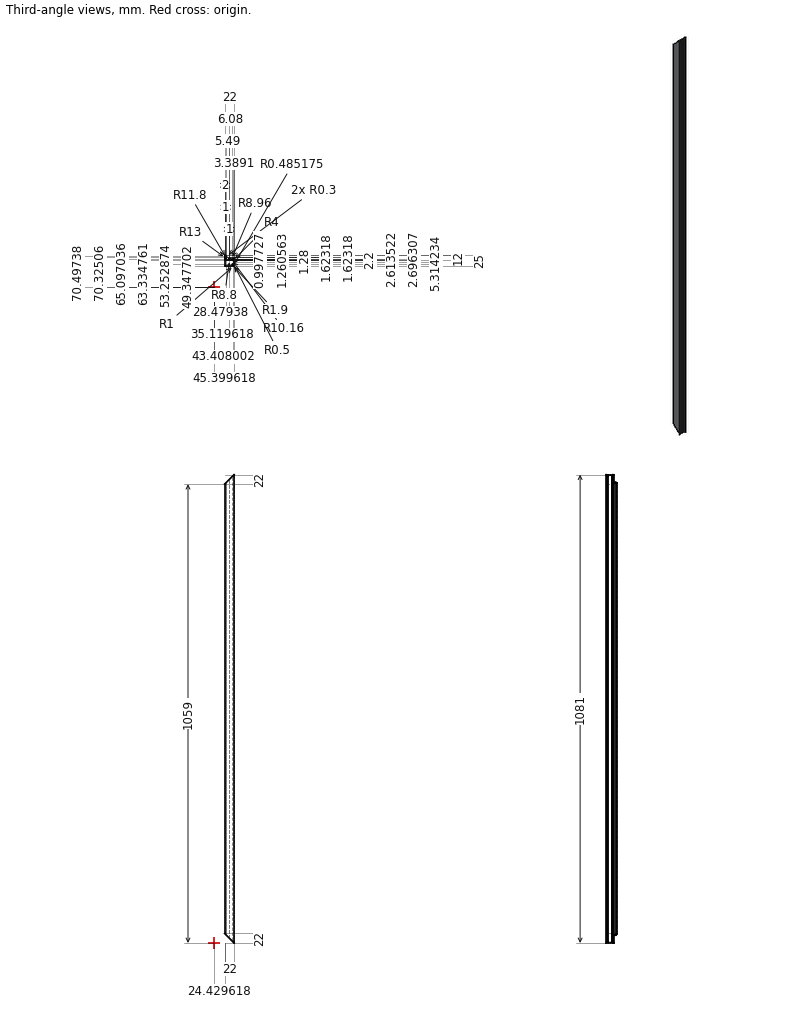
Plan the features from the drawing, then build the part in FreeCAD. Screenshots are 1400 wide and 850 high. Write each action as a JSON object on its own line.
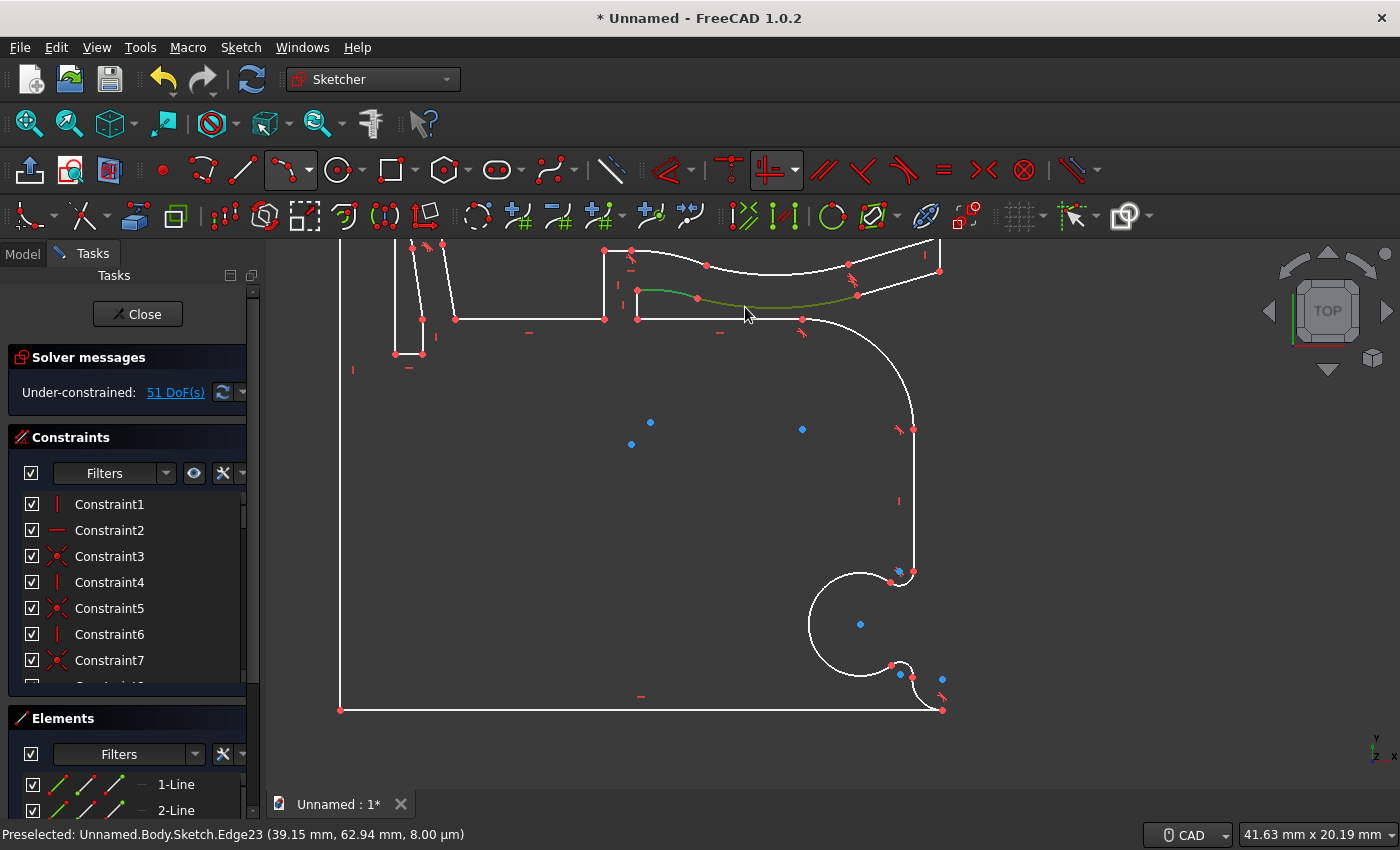
{"action": "left_click", "coordinate": [904, 170]}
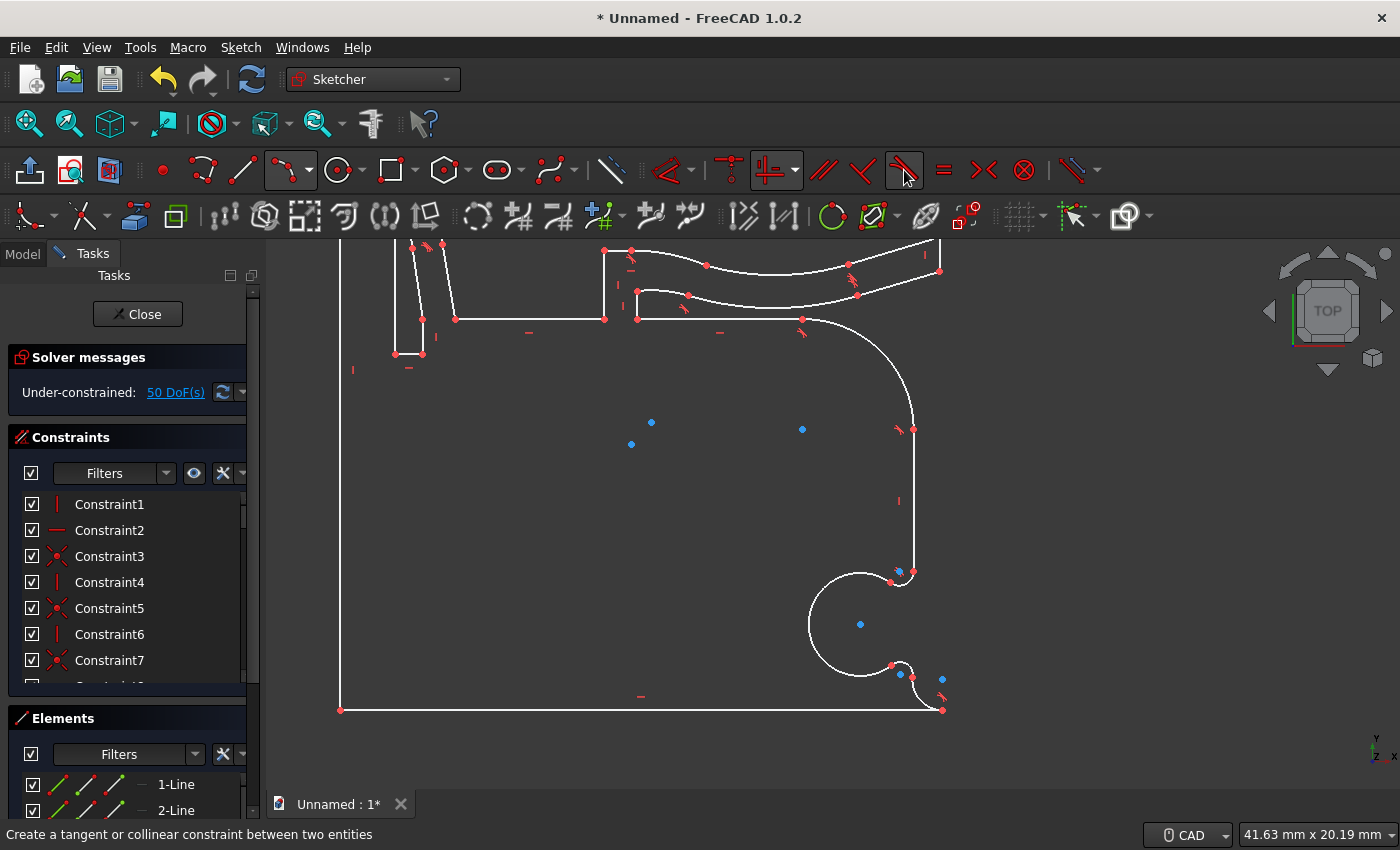
{"action": "left_click", "coordinate": [749, 274]}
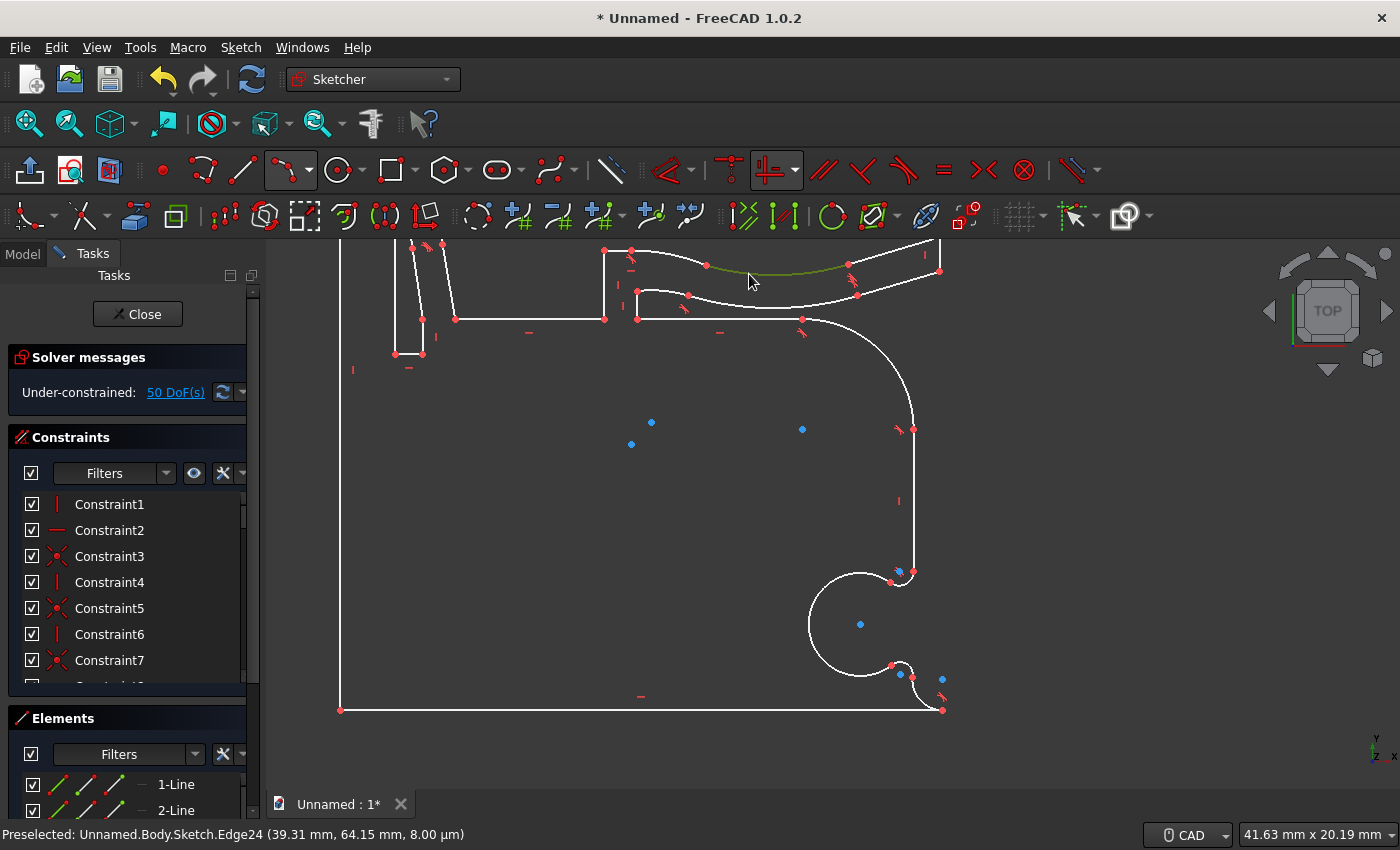
{"action": "scroll", "coordinate": [915, 692], "scroll_direction": "down", "scroll_amount": 3}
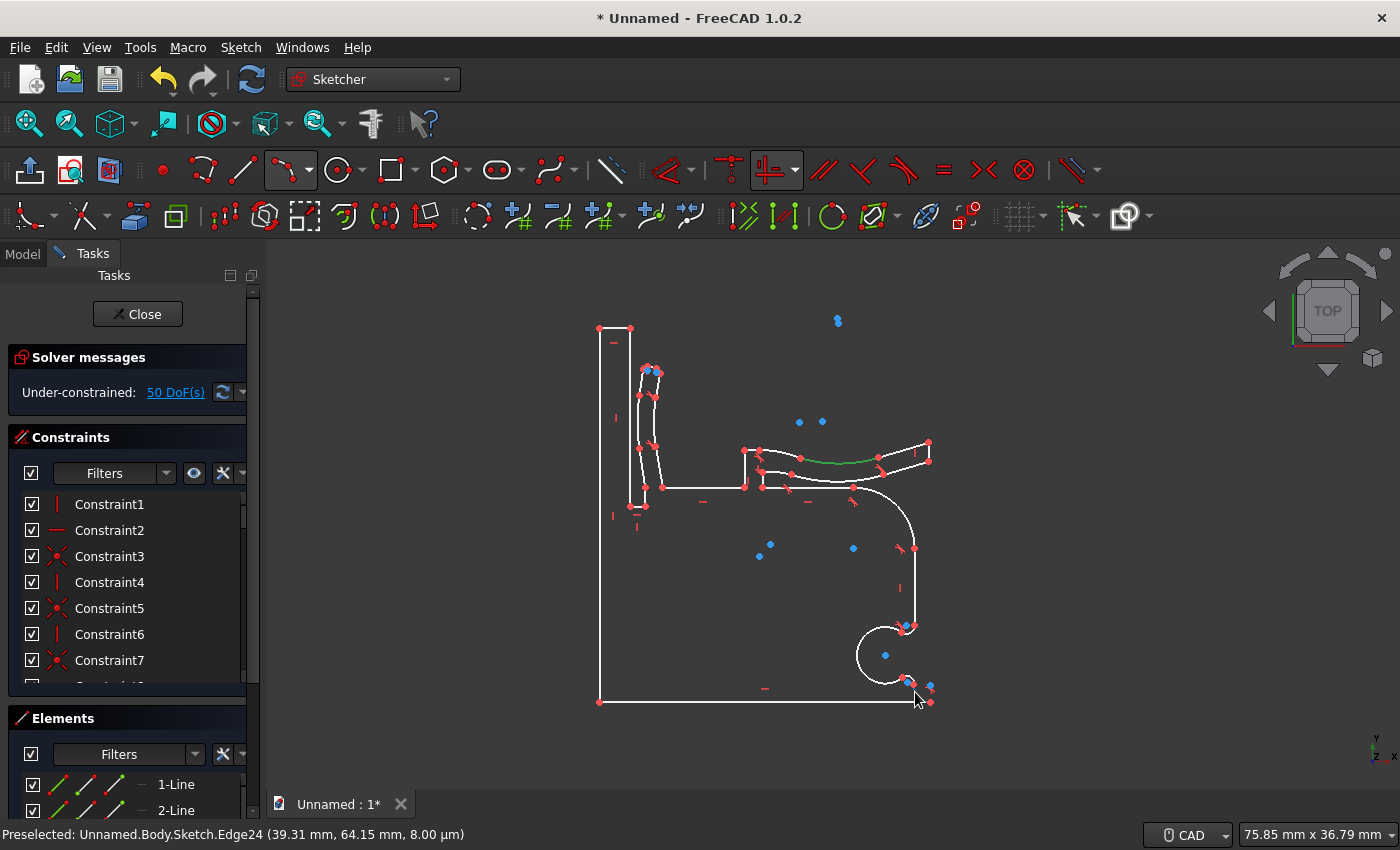
{"action": "left_click", "coordinate": [789, 454]}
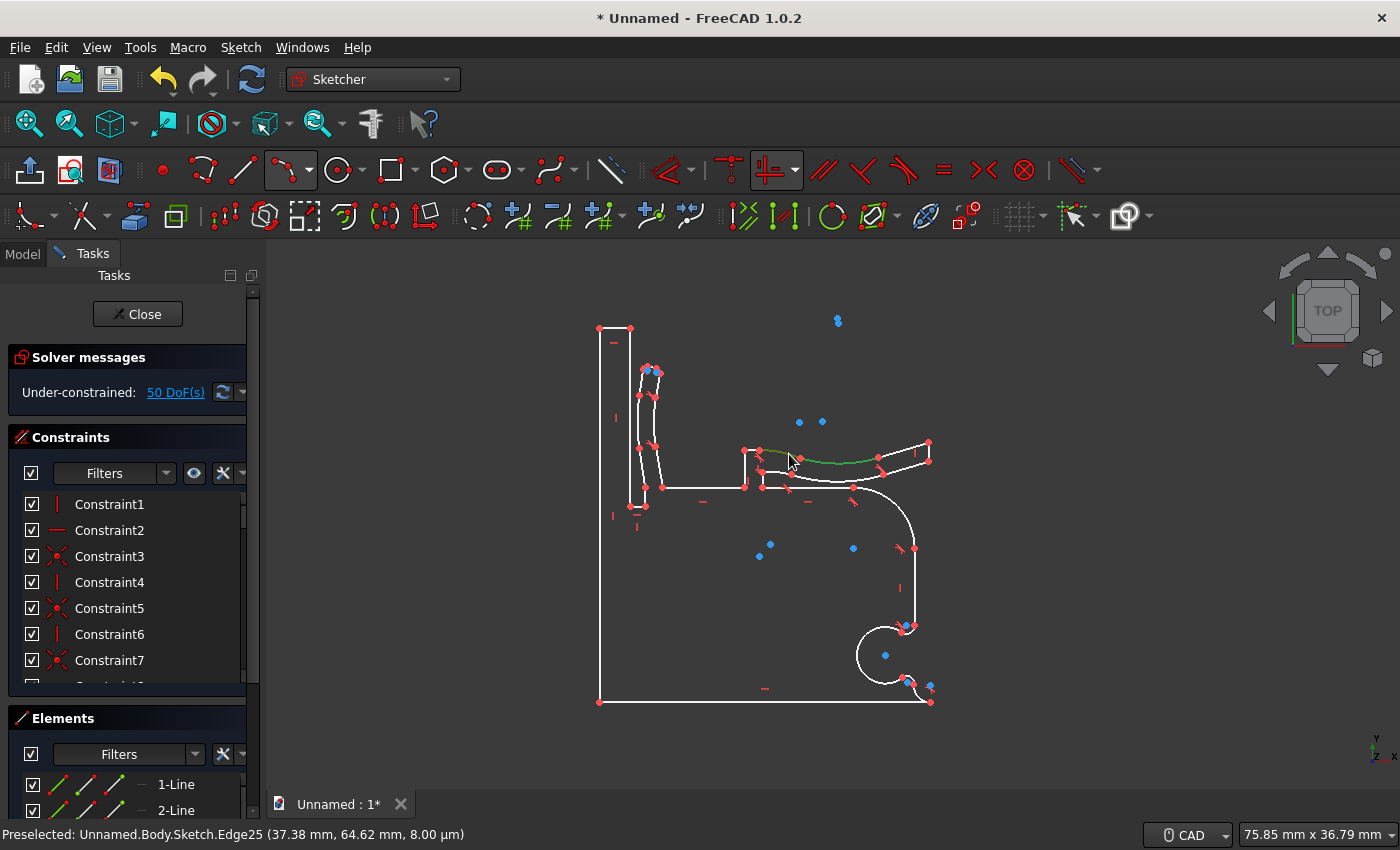
{"action": "left_click", "coordinate": [904, 170]}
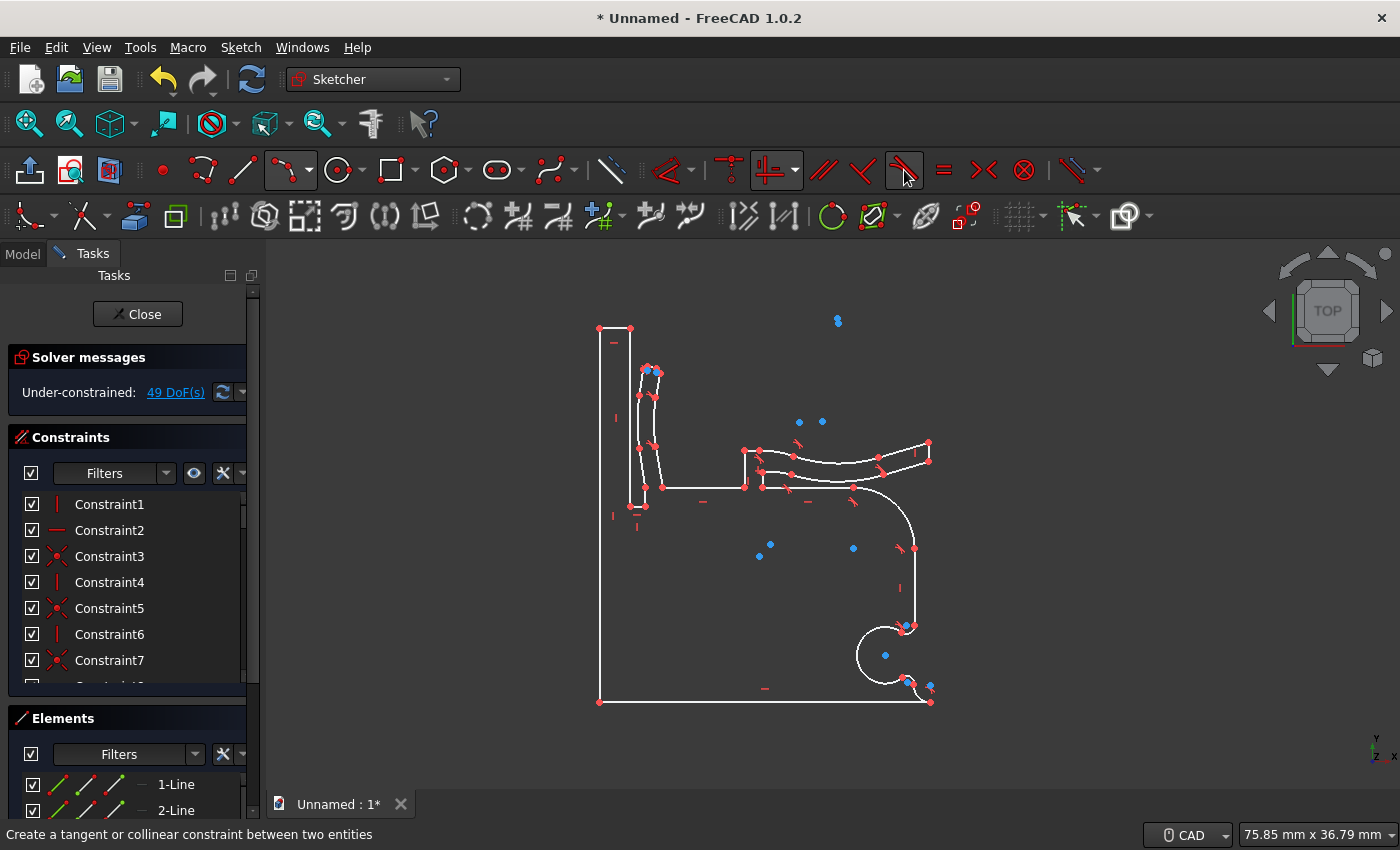
{"action": "scroll", "coordinate": [915, 693], "scroll_direction": "up", "scroll_amount": 3}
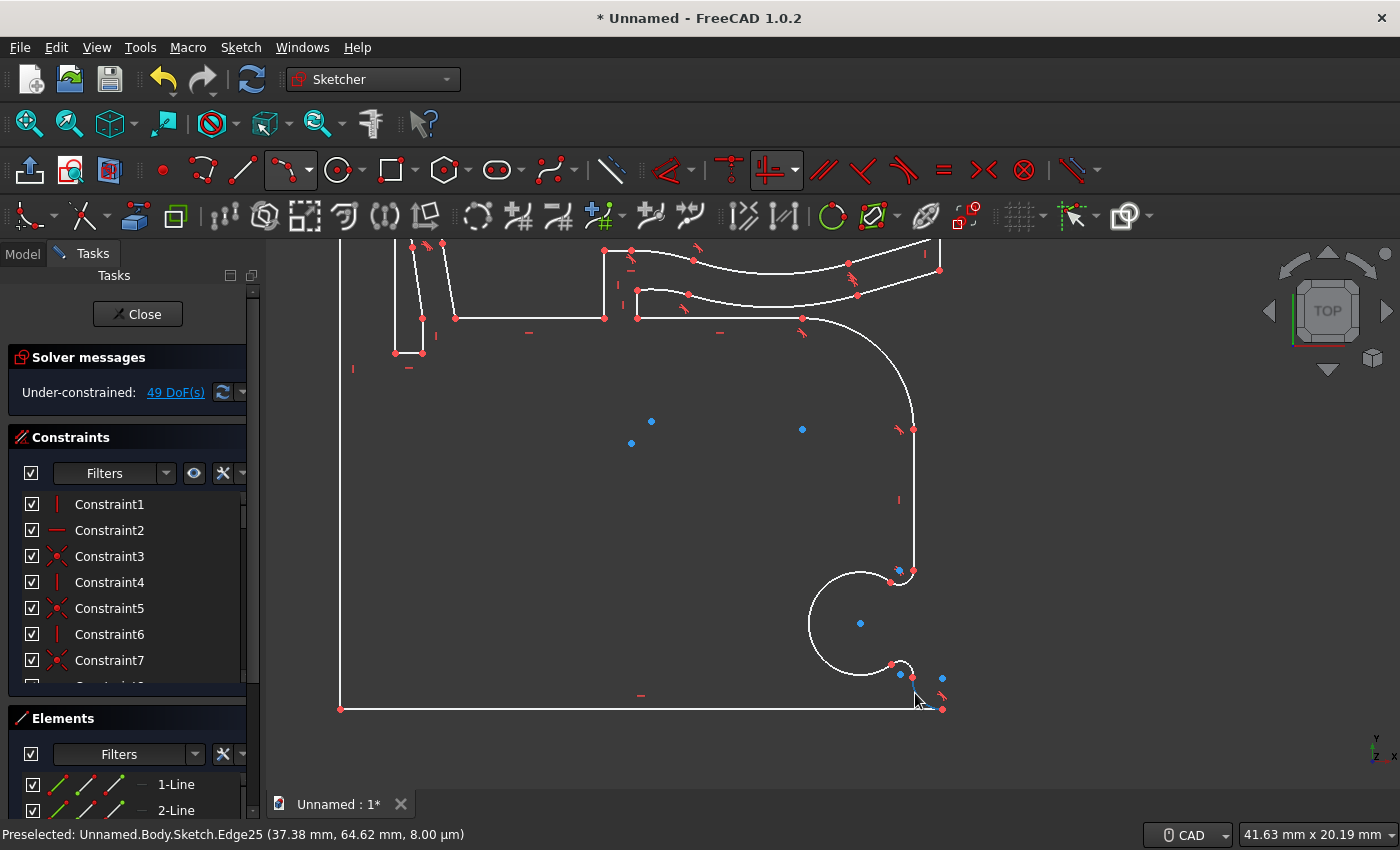
{"action": "left_click", "coordinate": [915, 692]}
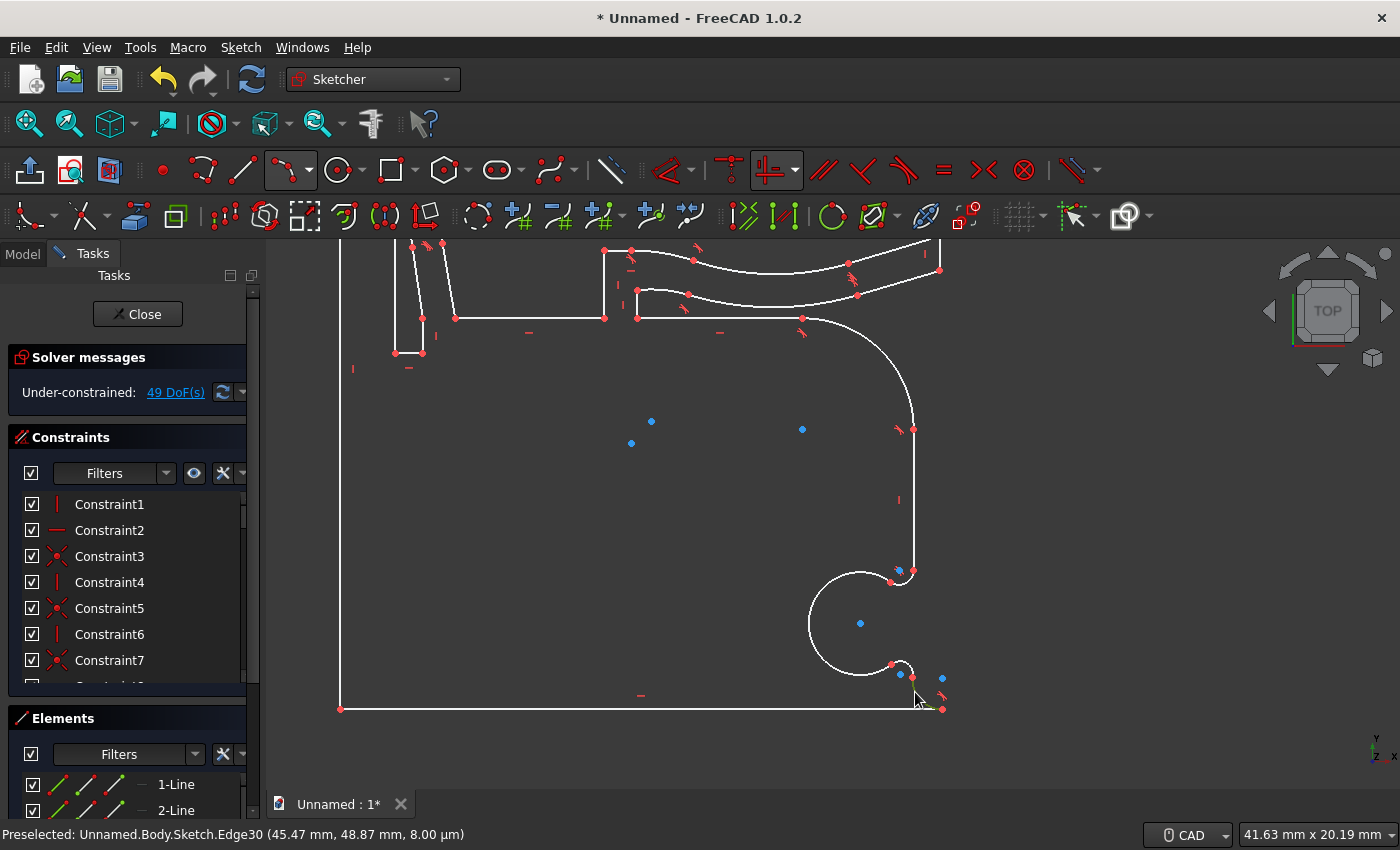
{"action": "scroll", "coordinate": [911, 668], "scroll_direction": "up", "scroll_amount": 2}